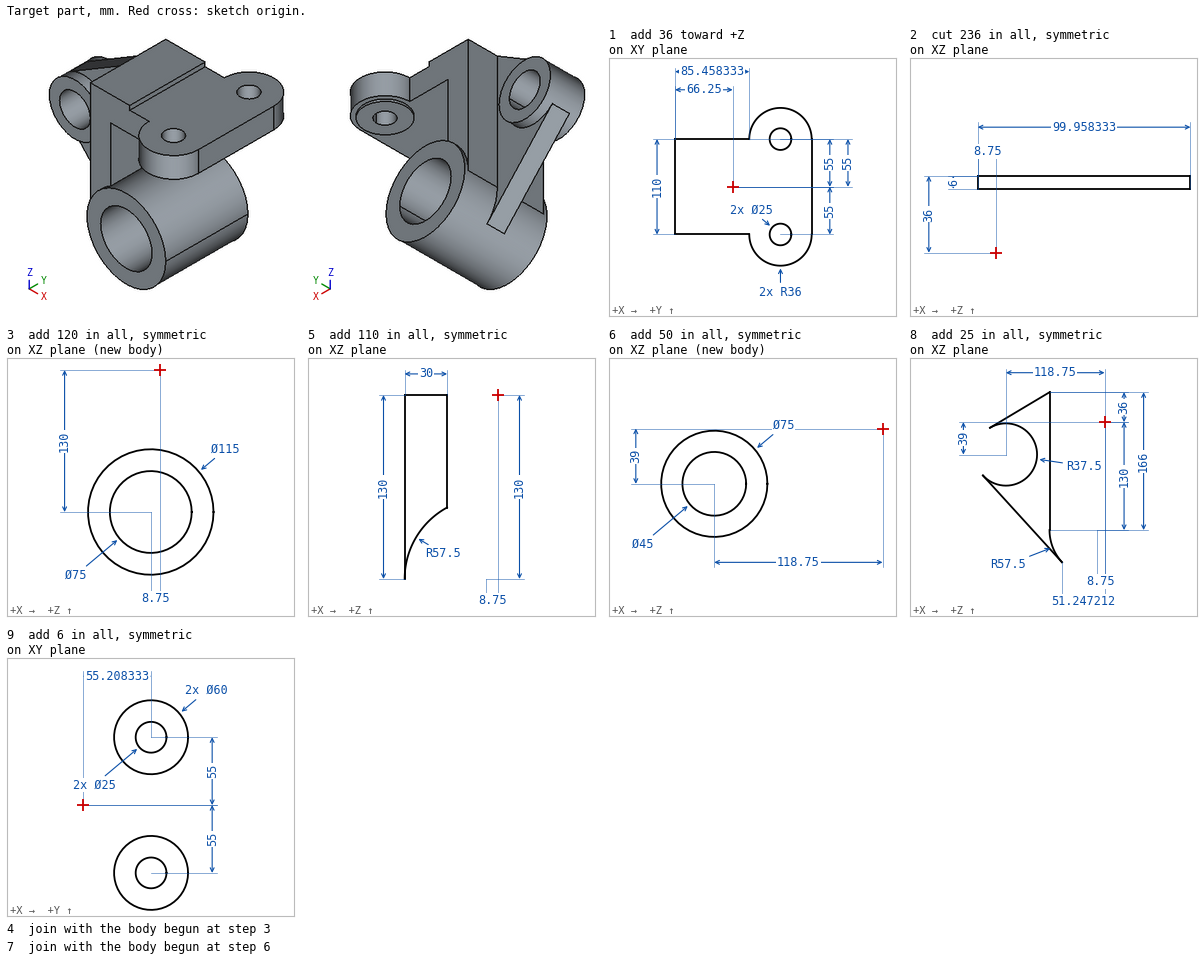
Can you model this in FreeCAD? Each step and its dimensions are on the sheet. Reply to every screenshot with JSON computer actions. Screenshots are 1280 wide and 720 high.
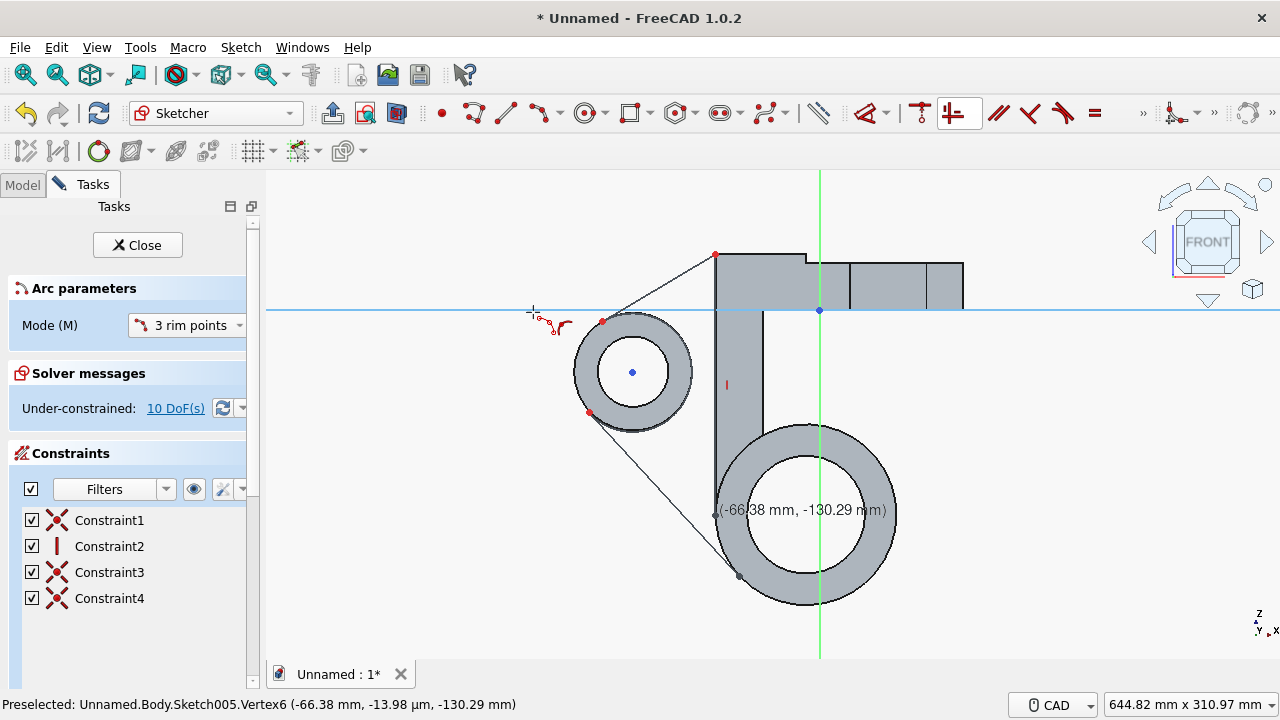
{"action": "left_click", "coordinate": [739, 577]}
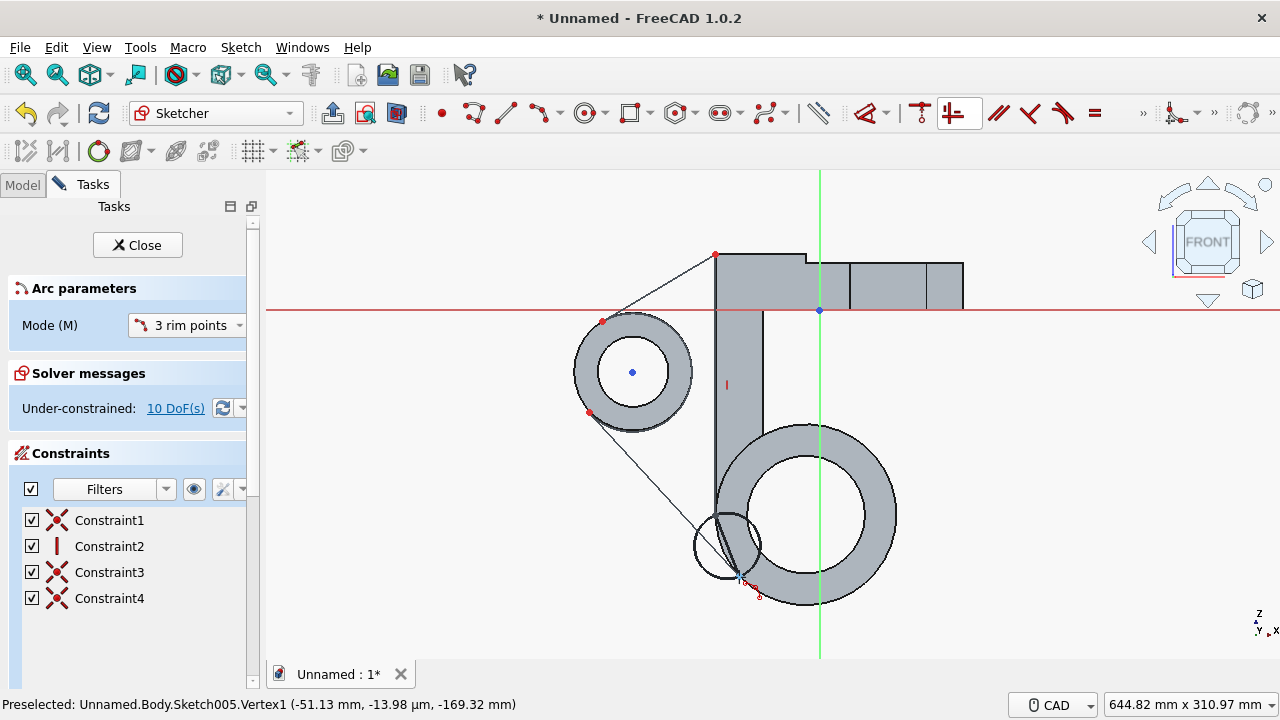
{"action": "scroll", "coordinate": [722, 547], "scroll_direction": "up", "scroll_amount": 5}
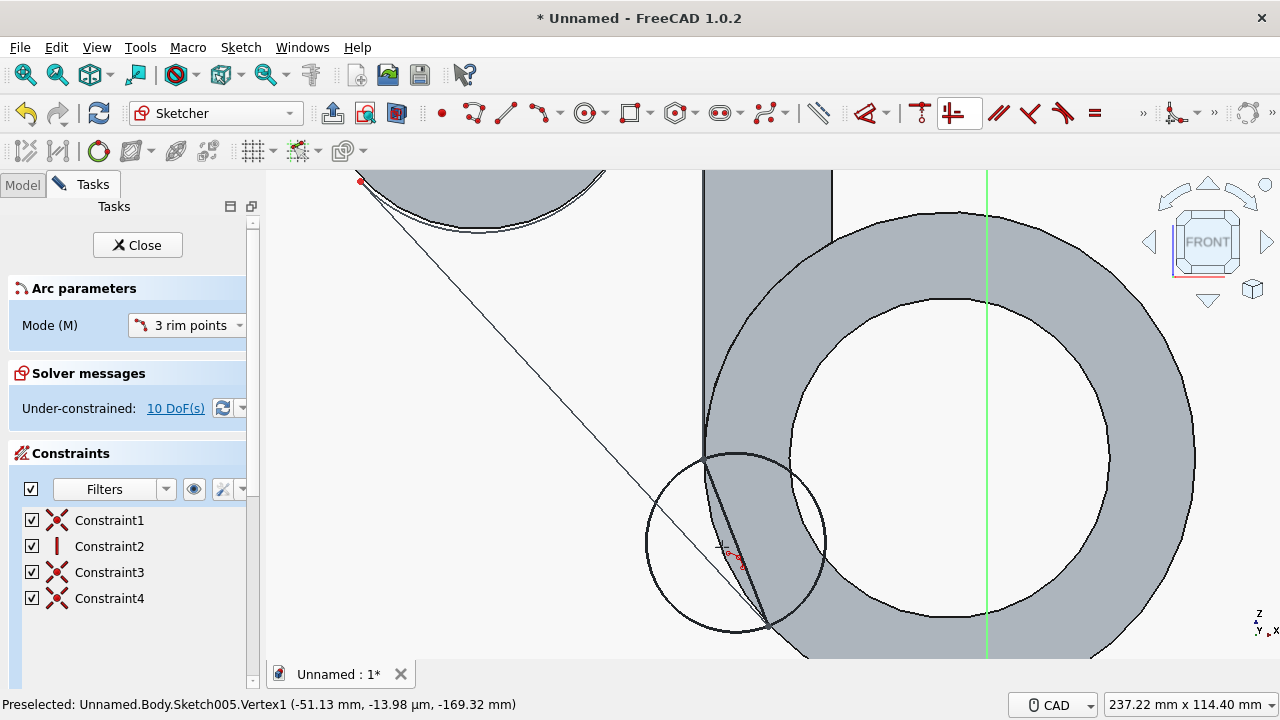
{"action": "left_click", "coordinate": [720, 547]}
{"action": "key", "text": "Escape"}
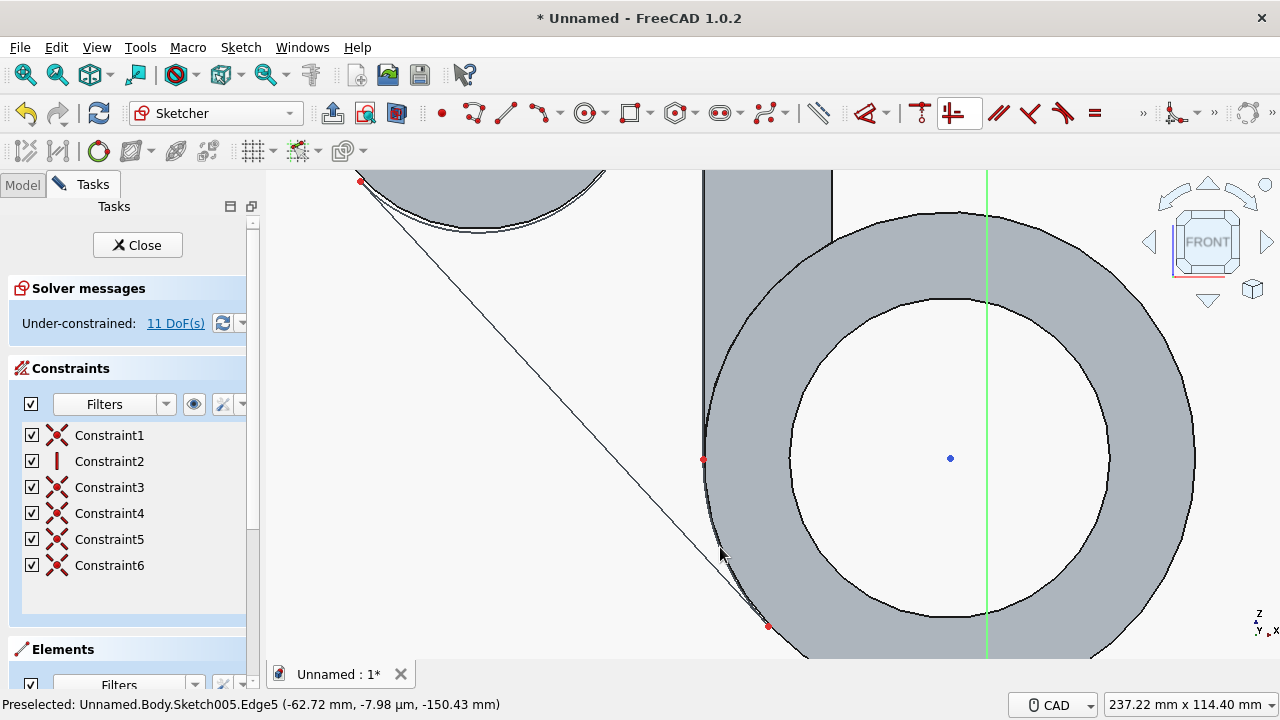
{"action": "left_click", "coordinate": [646, 493]}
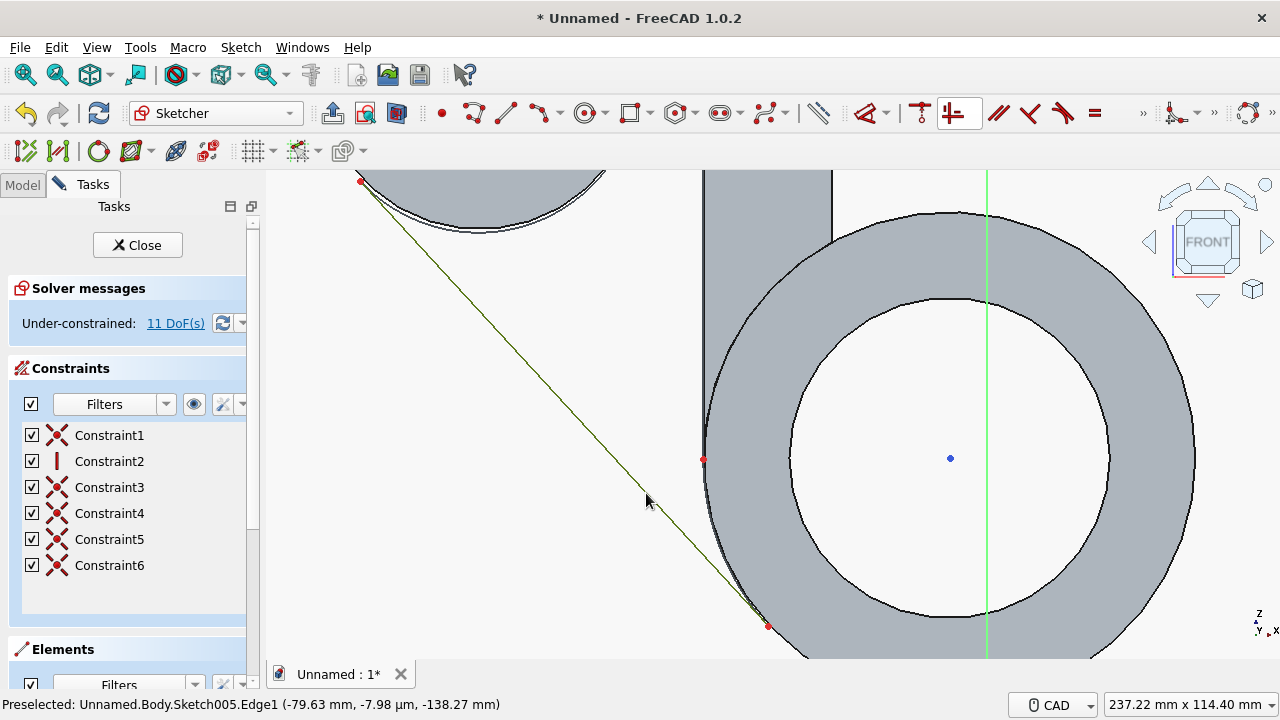
{"action": "left_click", "coordinate": [559, 211]}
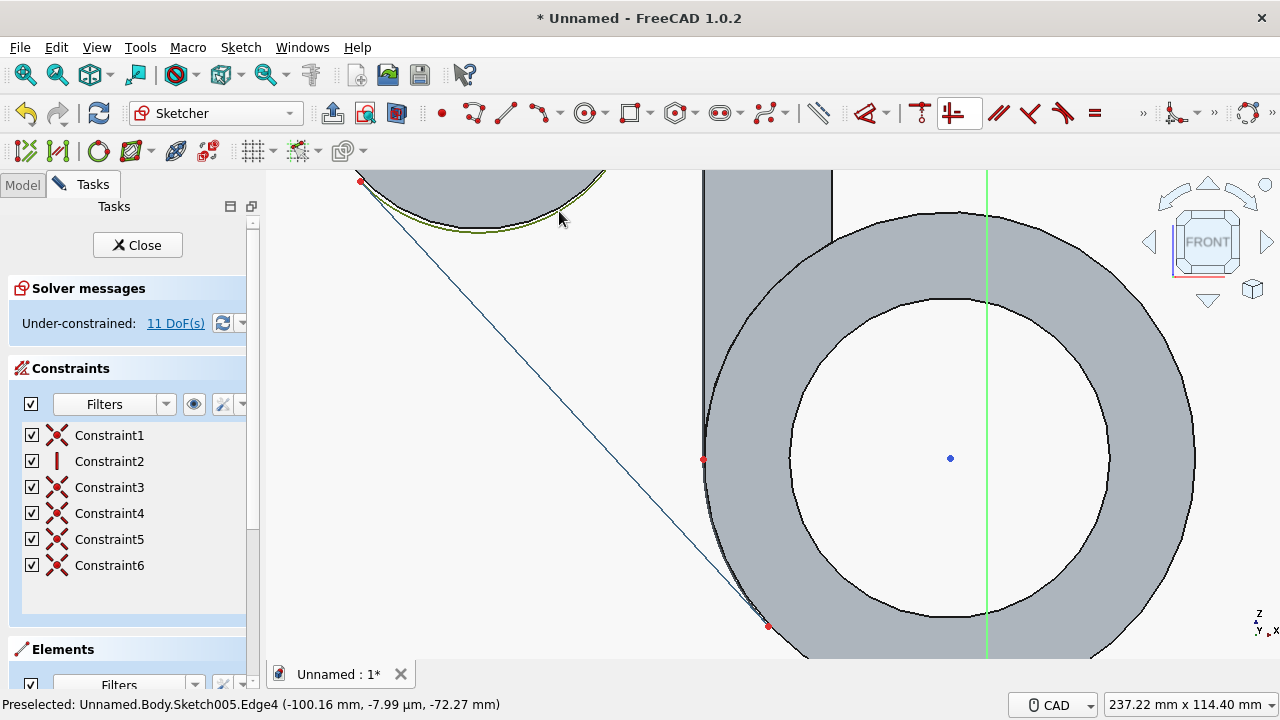
{"action": "left_click", "coordinate": [1064, 114]}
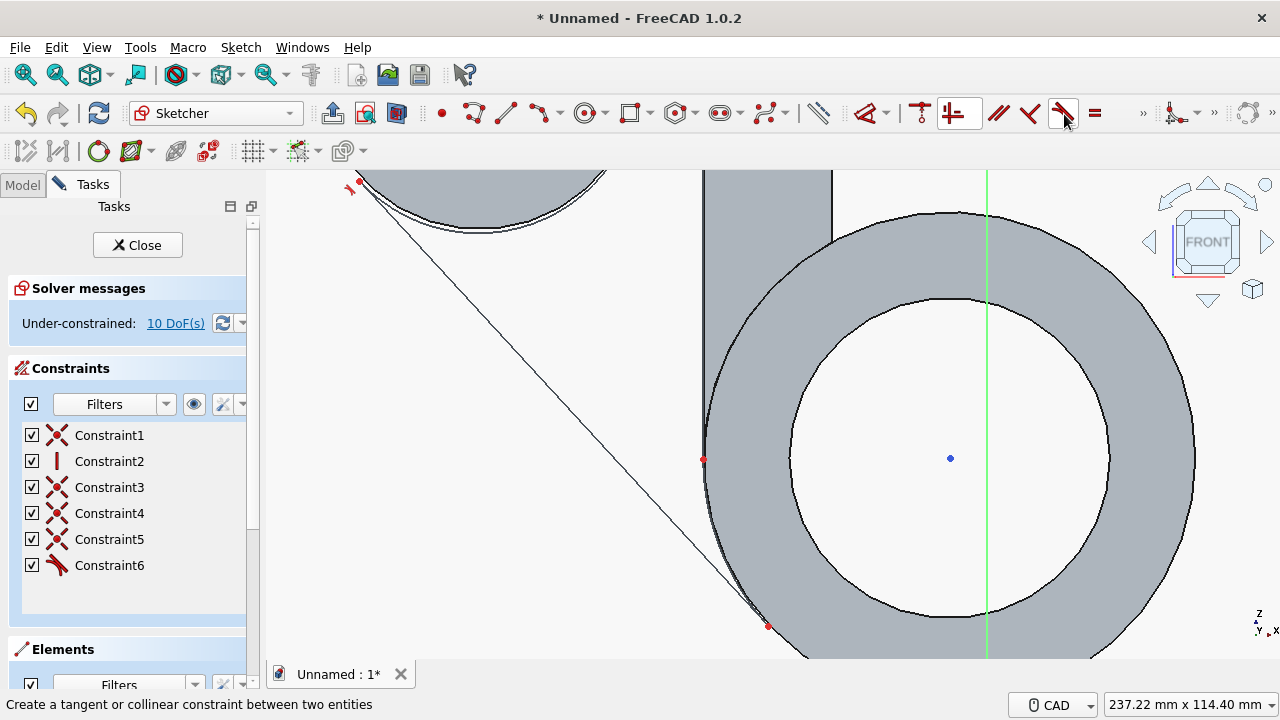
{"action": "scroll", "coordinate": [722, 547], "scroll_direction": "down", "scroll_amount": 5}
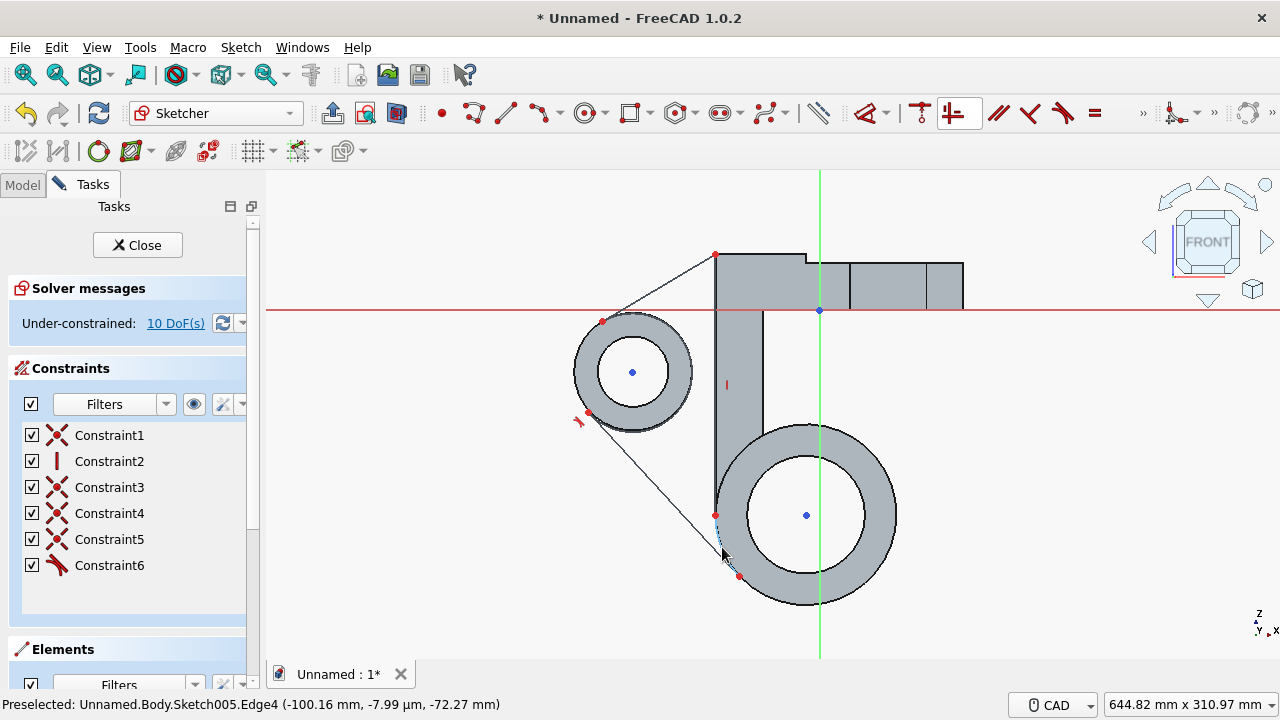
{"action": "scroll", "coordinate": [637, 301], "scroll_direction": "up", "scroll_amount": 3}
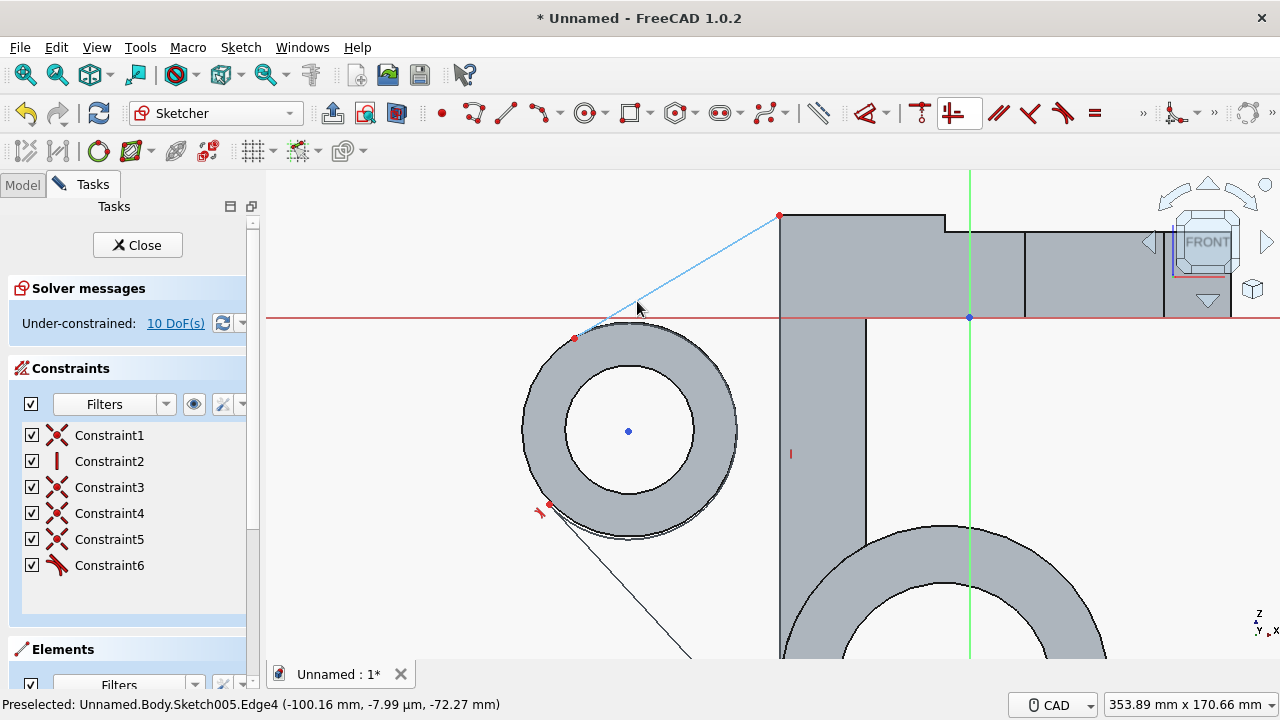
{"action": "left_click", "coordinate": [636, 301]}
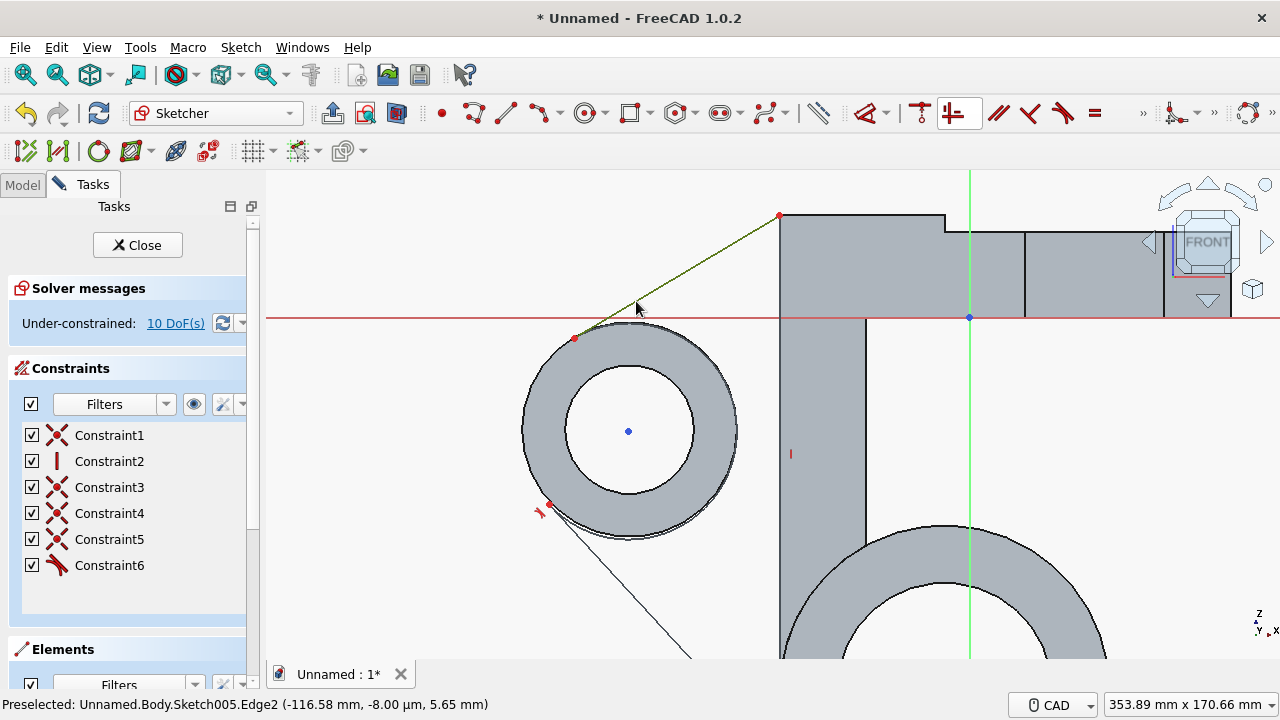
{"action": "left_click", "coordinate": [683, 525]}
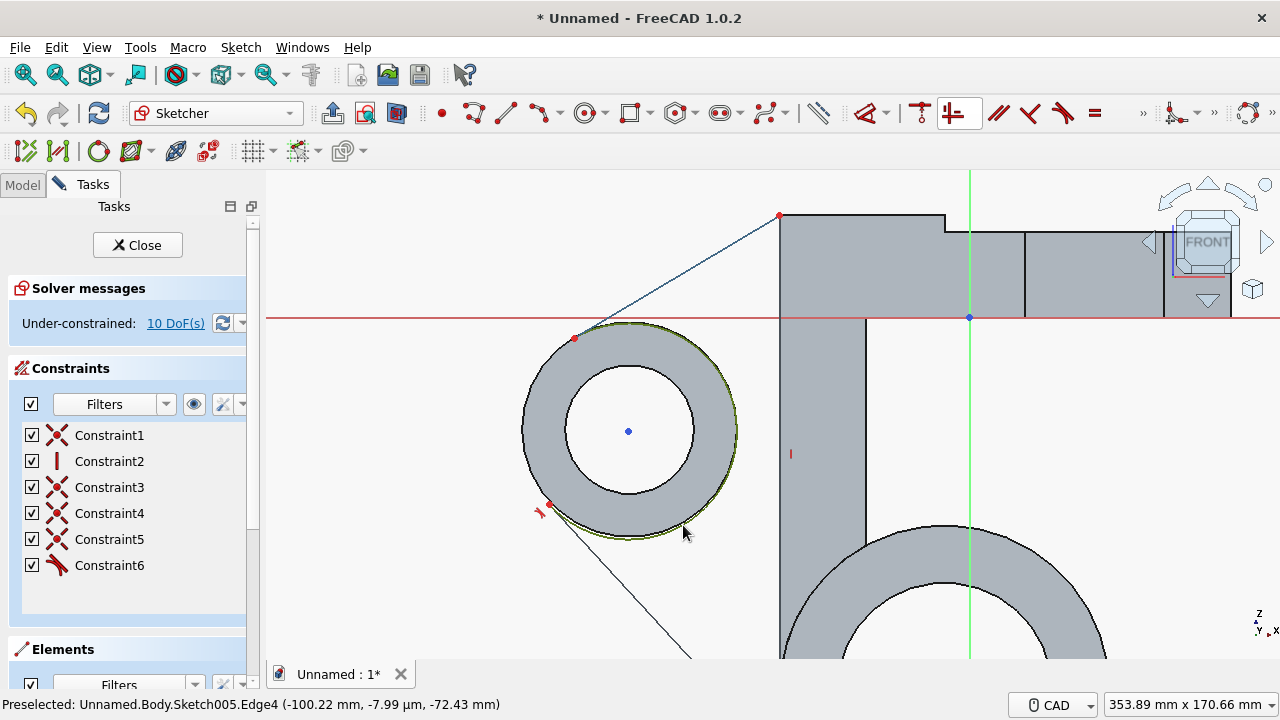
{"action": "left_click", "coordinate": [1064, 114]}